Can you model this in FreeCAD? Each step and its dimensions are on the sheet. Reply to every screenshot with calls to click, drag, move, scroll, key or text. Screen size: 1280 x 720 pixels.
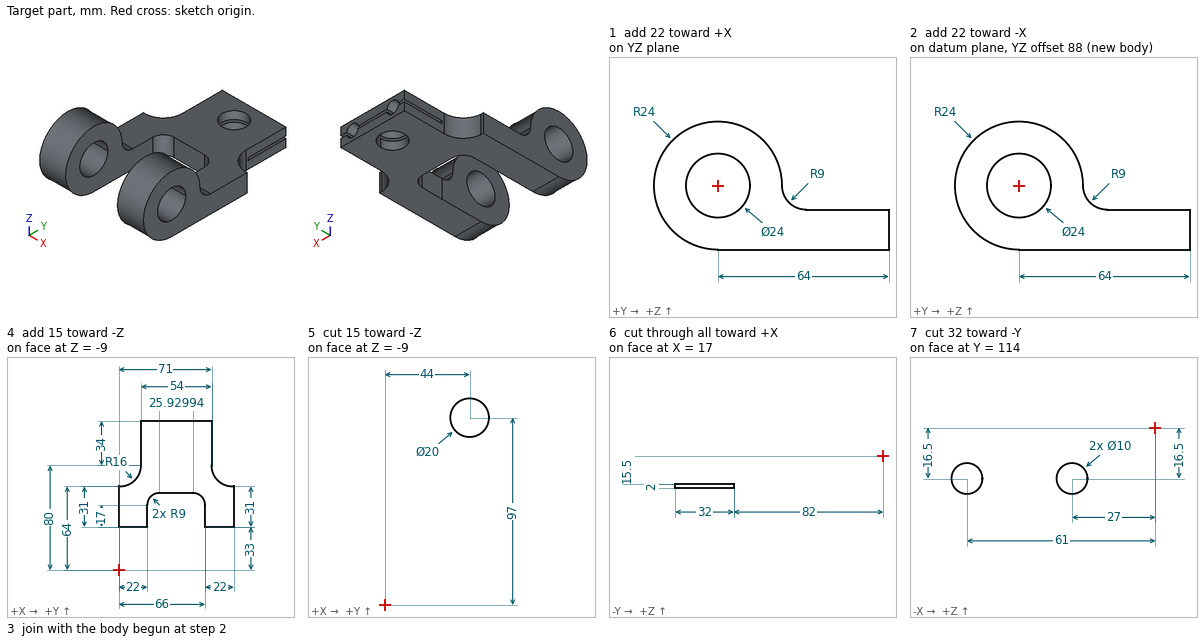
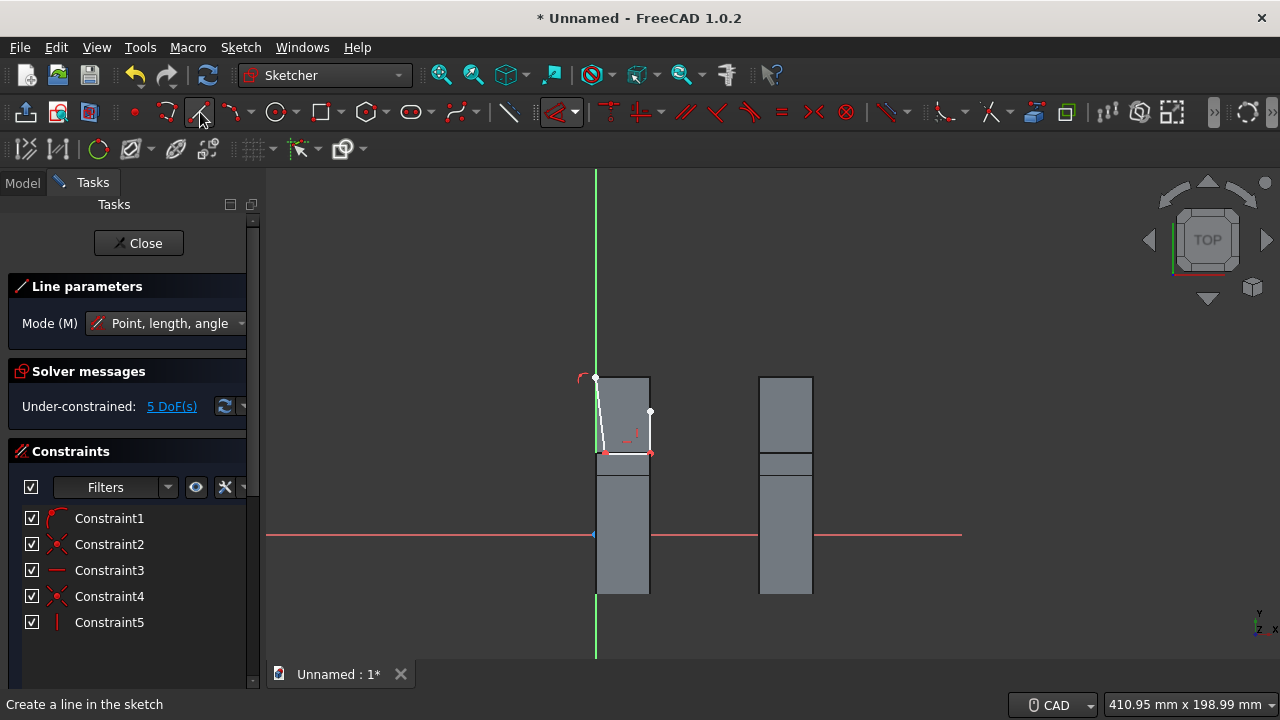
click(672, 389)
click(736, 389)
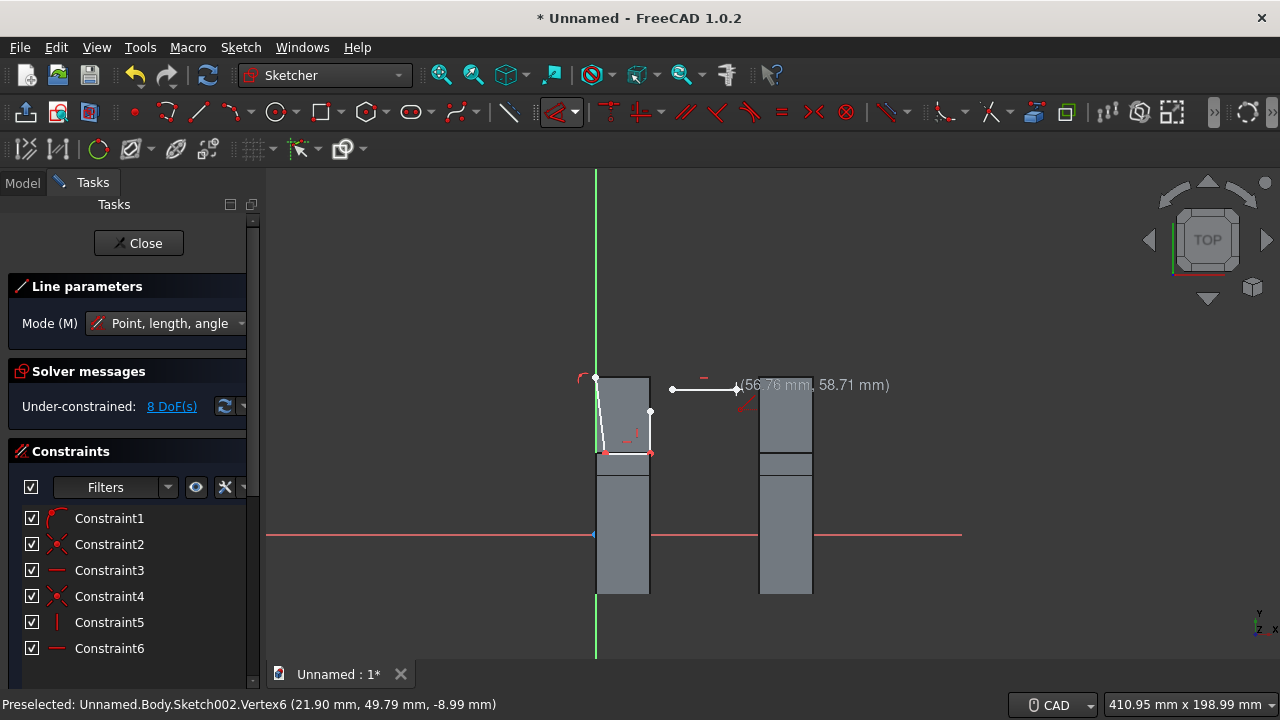
click(168, 112)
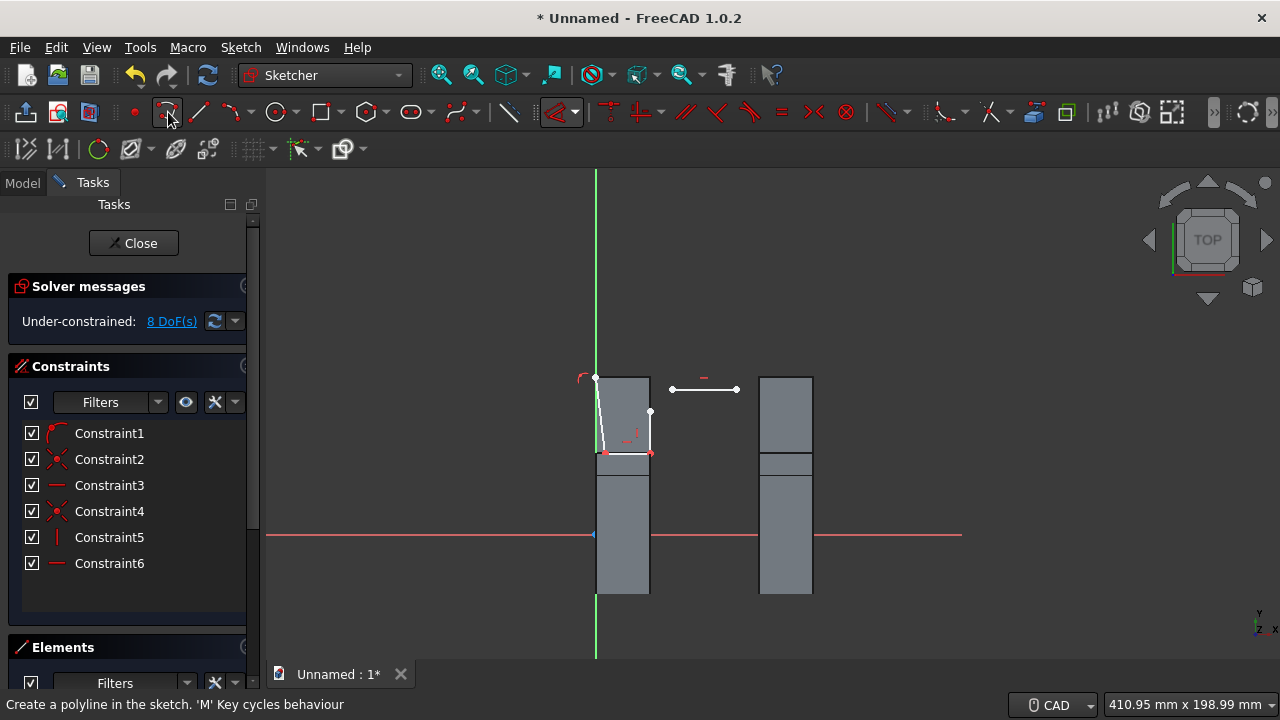
click(759, 411)
click(762, 453)
click(813, 453)
click(813, 377)
right_click(813, 377)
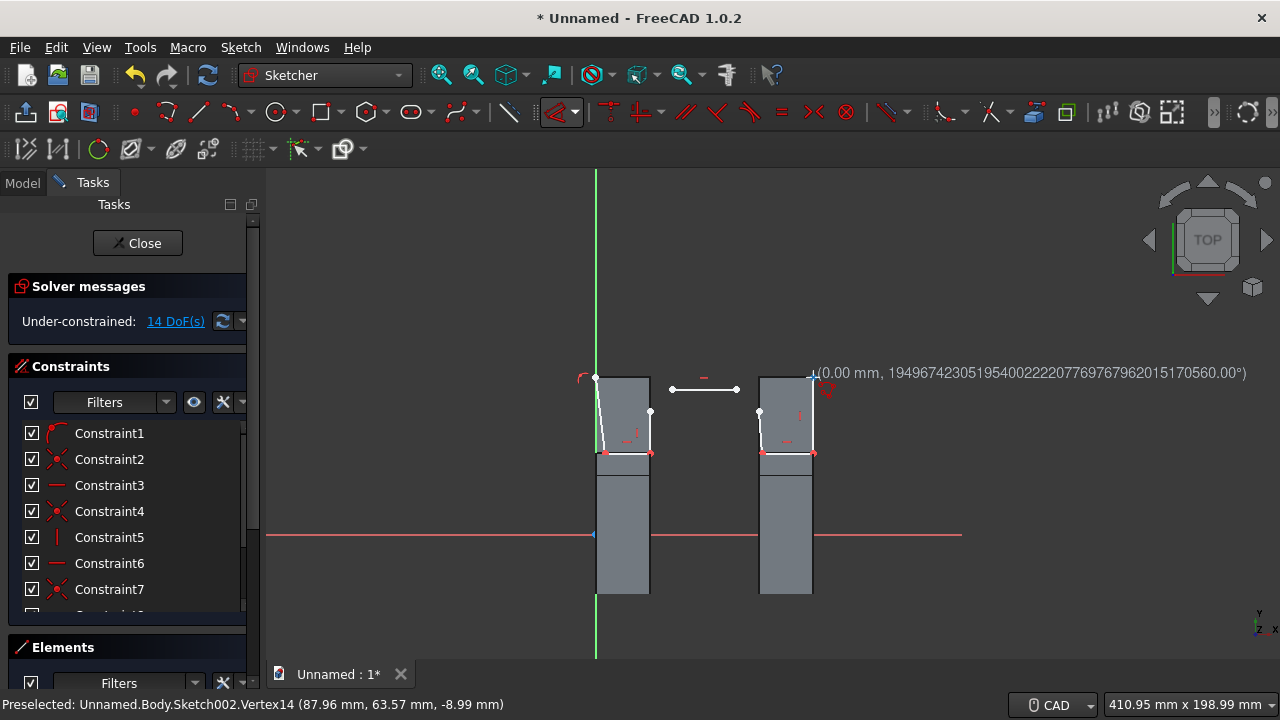
click(771, 338)
click(771, 254)
click(638, 254)
click(638, 337)
right_click(638, 337)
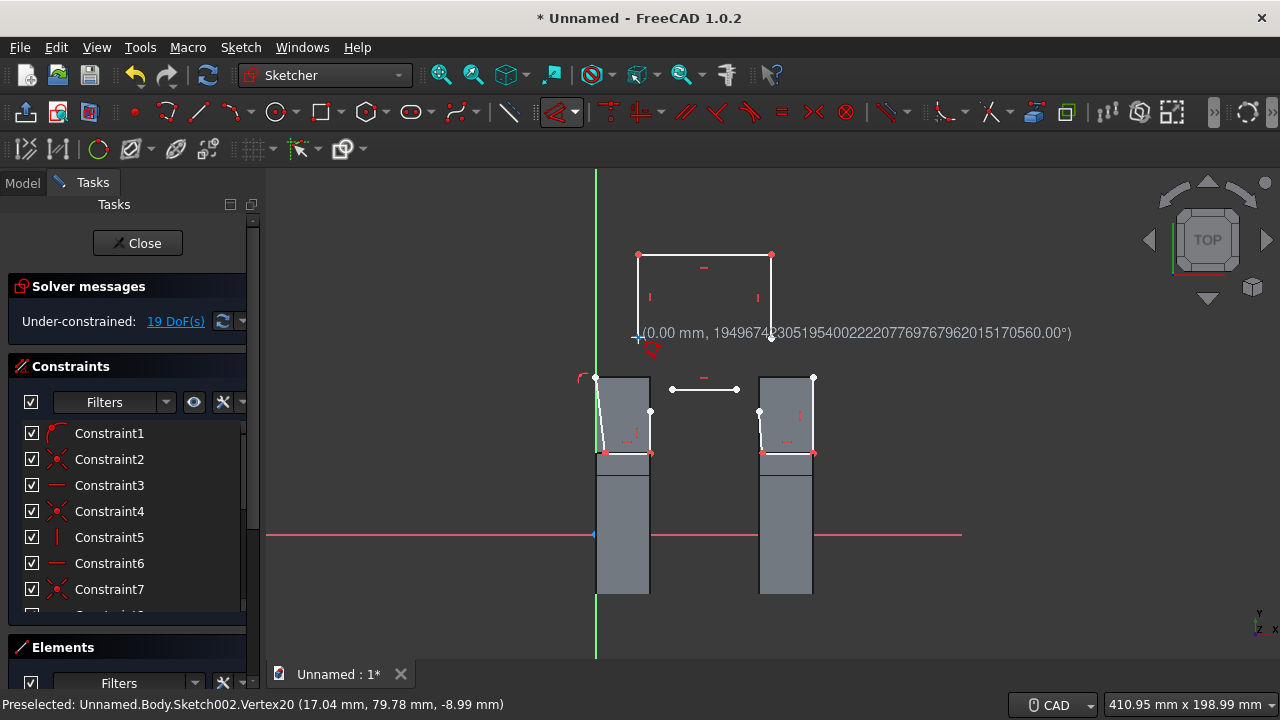
click(232, 112)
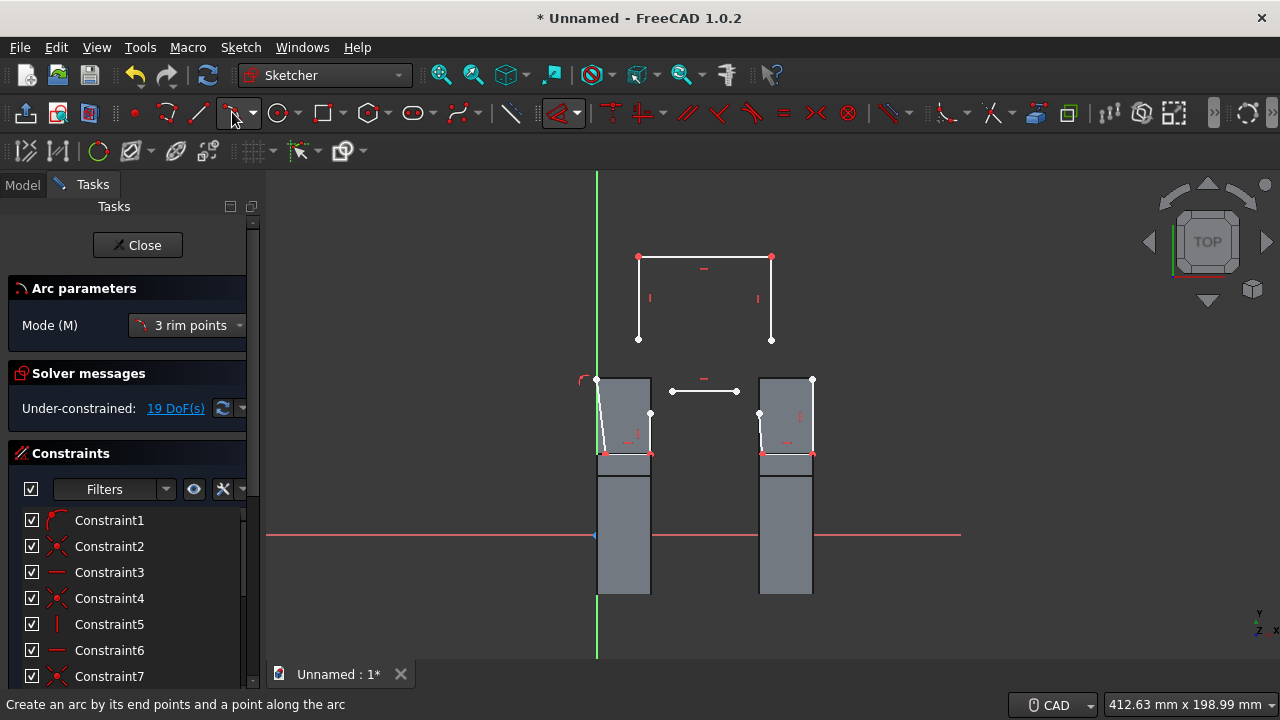
click(651, 413)
click(672, 391)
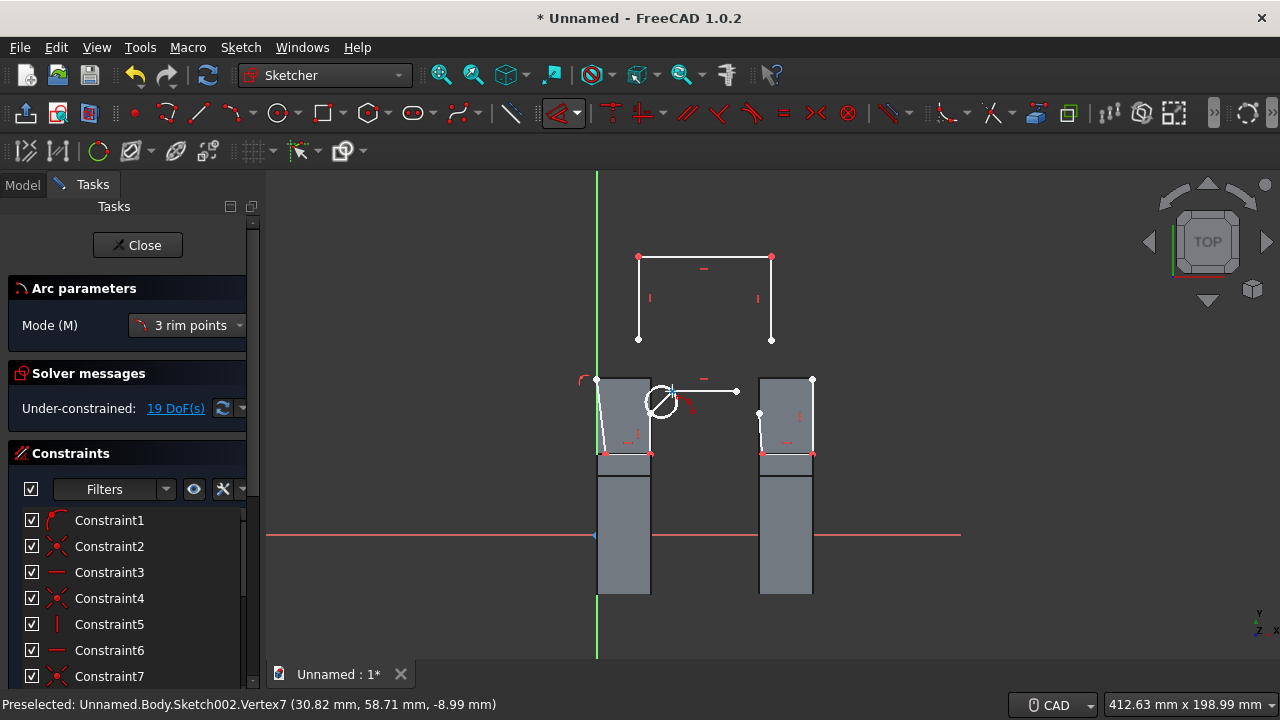
scroll(657, 397, up, 5)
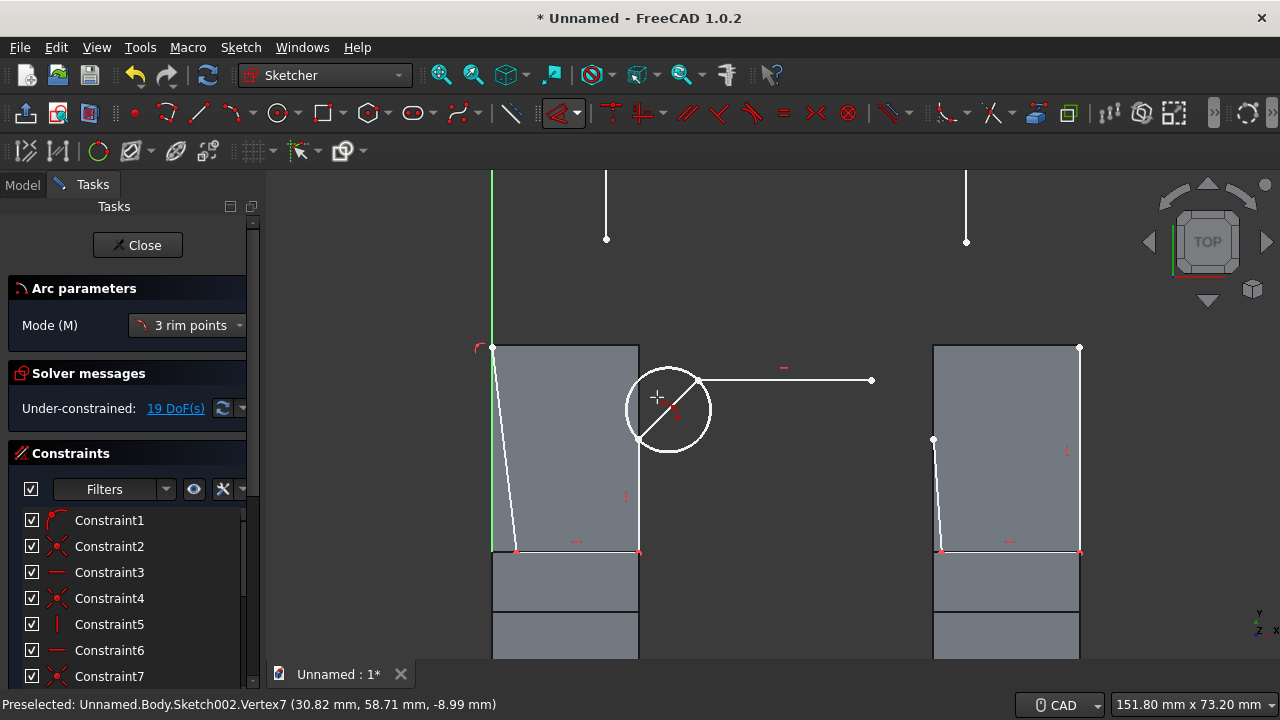
click(657, 396)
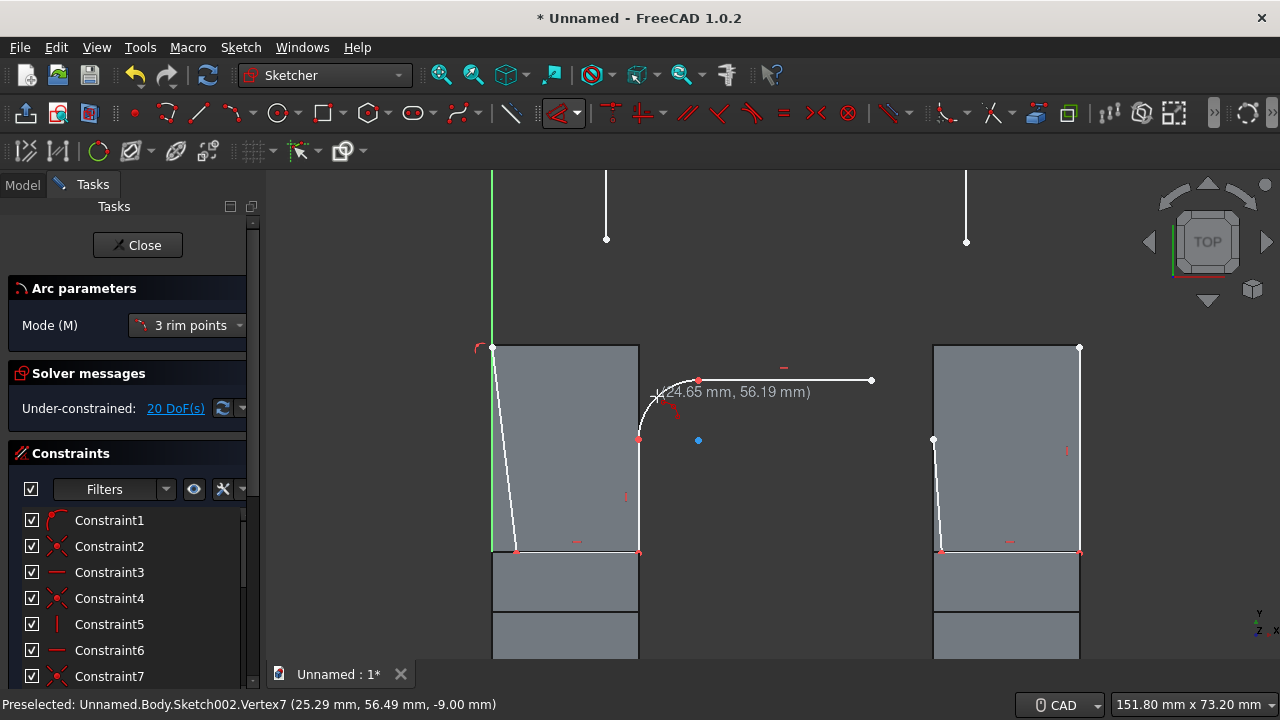
click(871, 380)
click(934, 440)
click(915, 396)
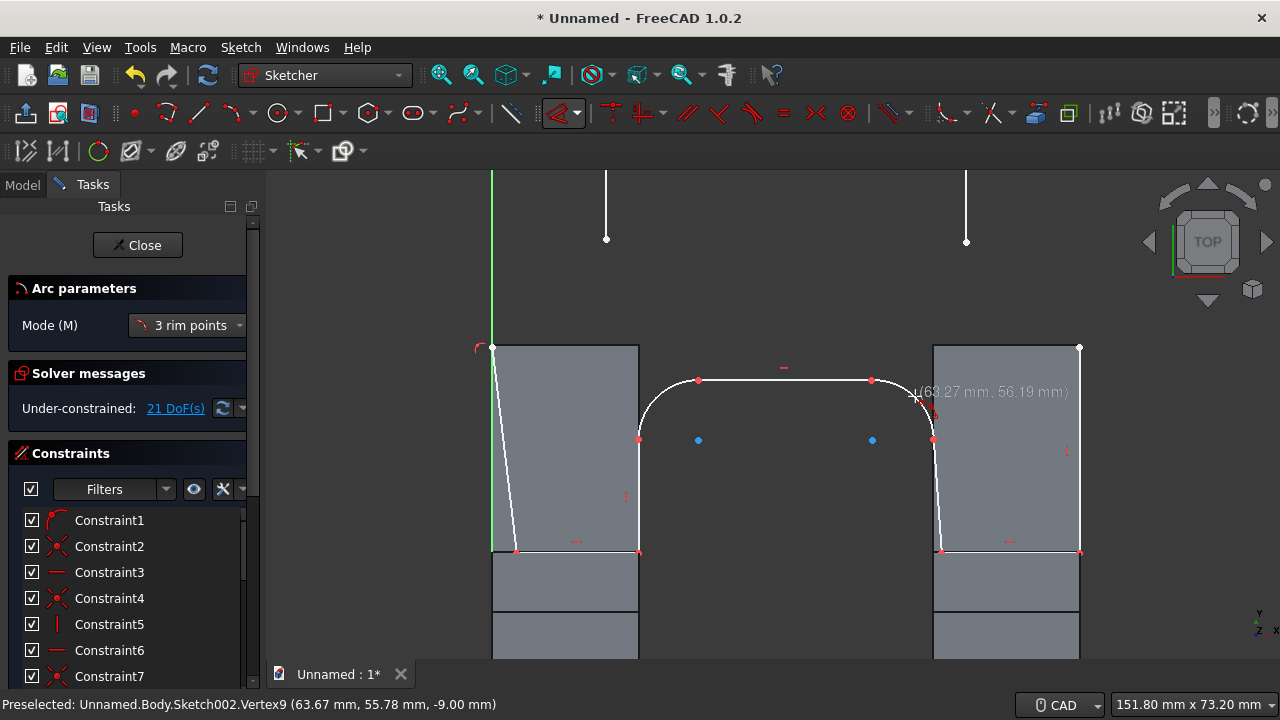
click(1080, 348)
click(966, 242)
click(1000, 316)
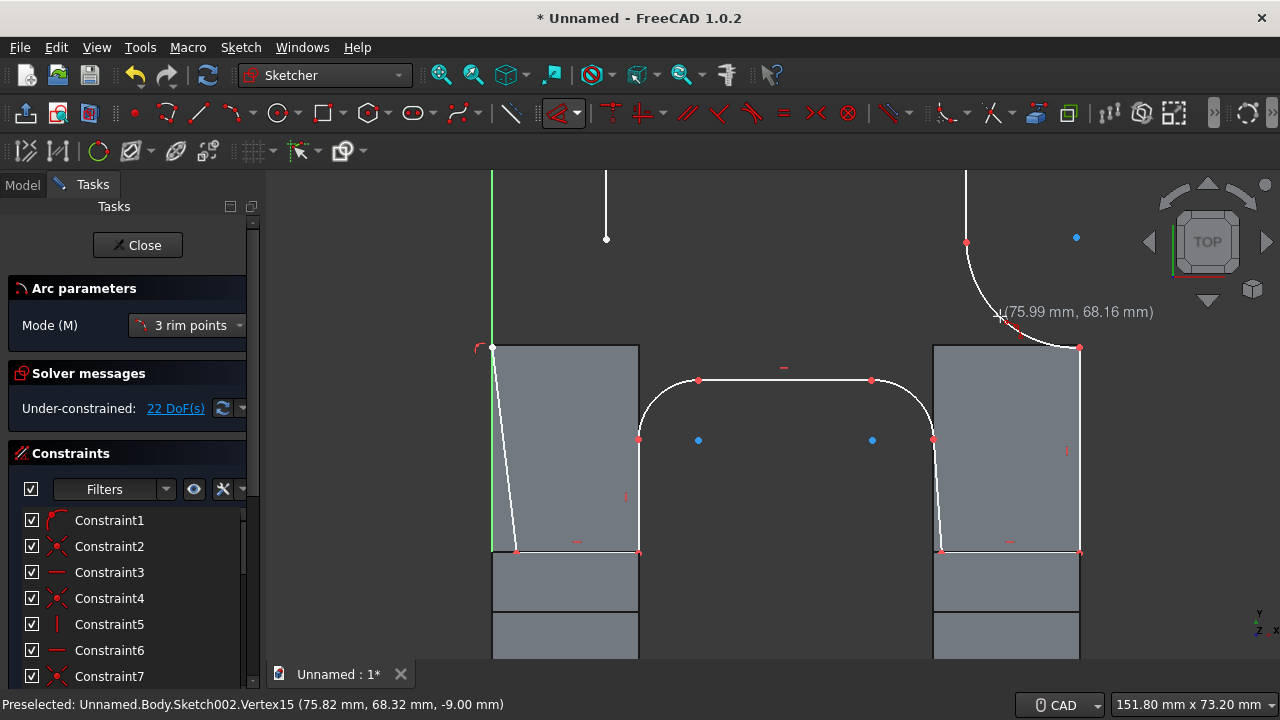
click(606, 239)
click(492, 348)
click(572, 316)
key(Escape)